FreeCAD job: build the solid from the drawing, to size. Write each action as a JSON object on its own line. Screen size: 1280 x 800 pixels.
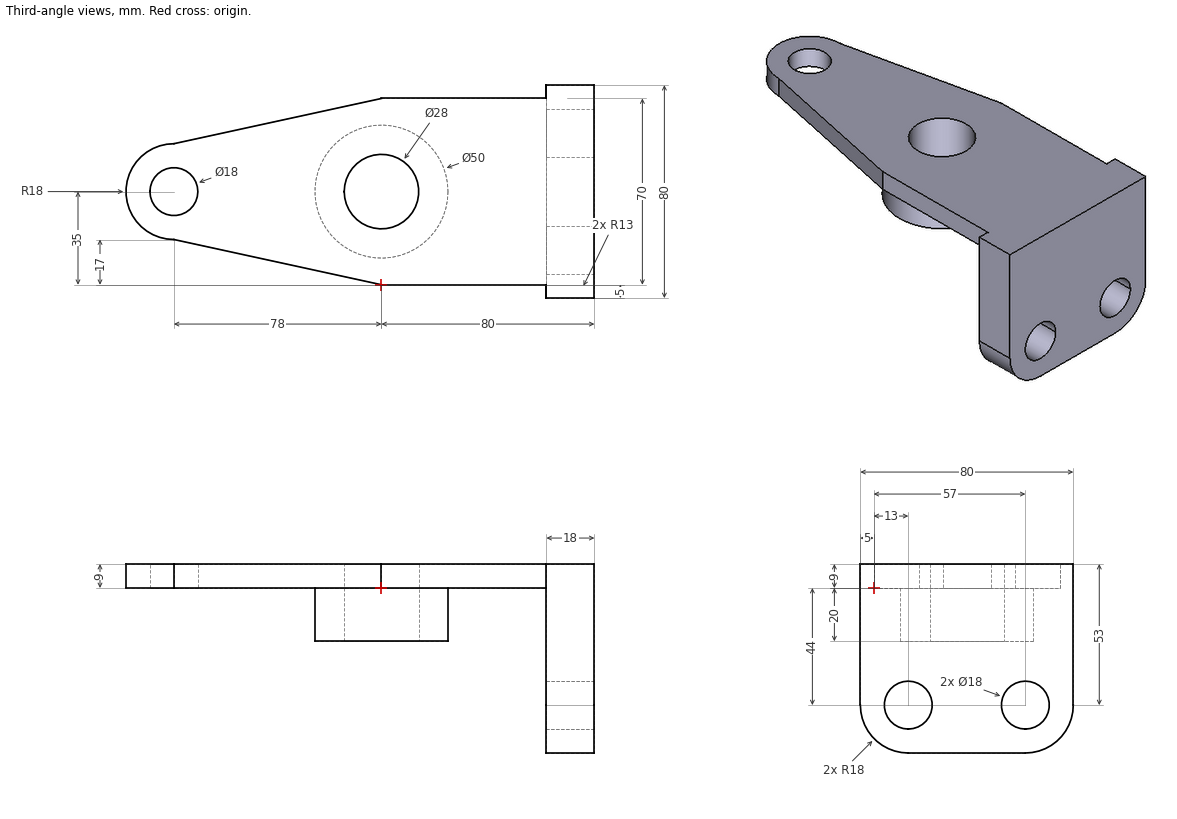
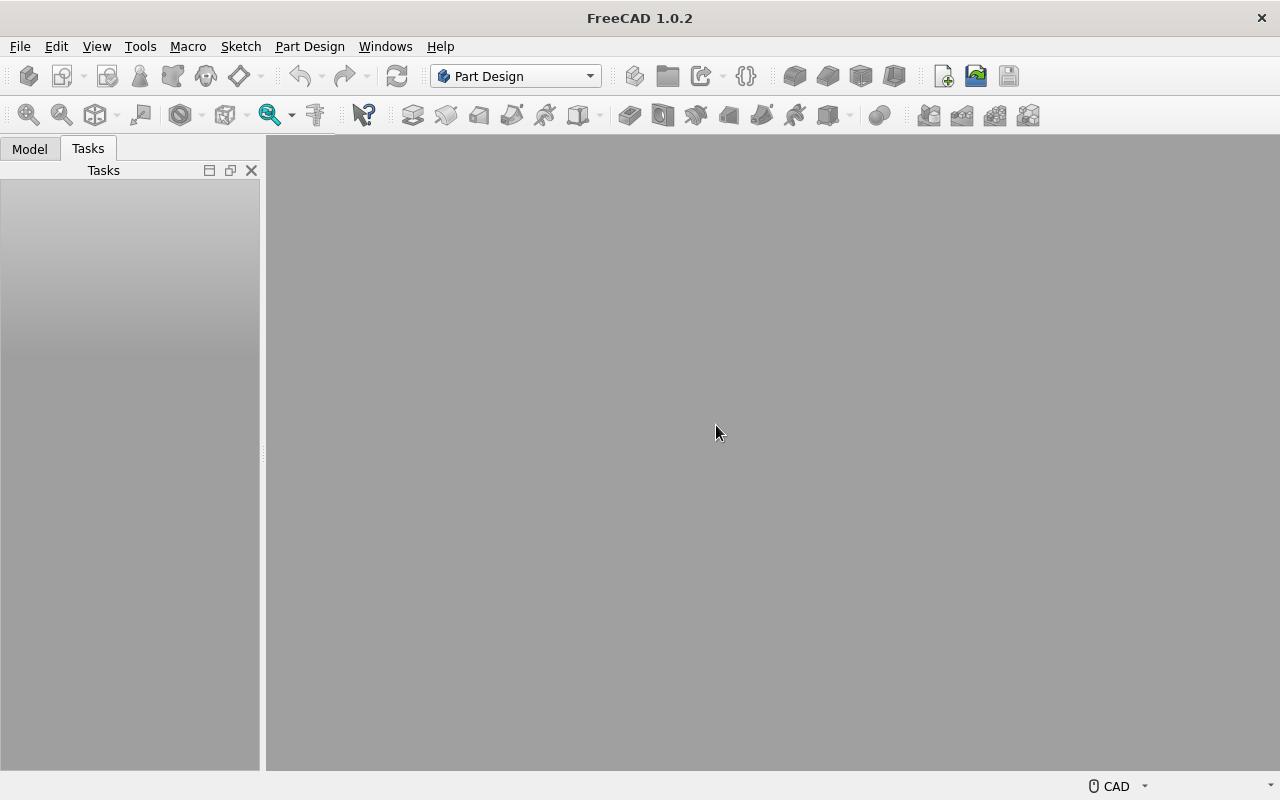
{"action": "left_click", "coordinate": [943, 76]}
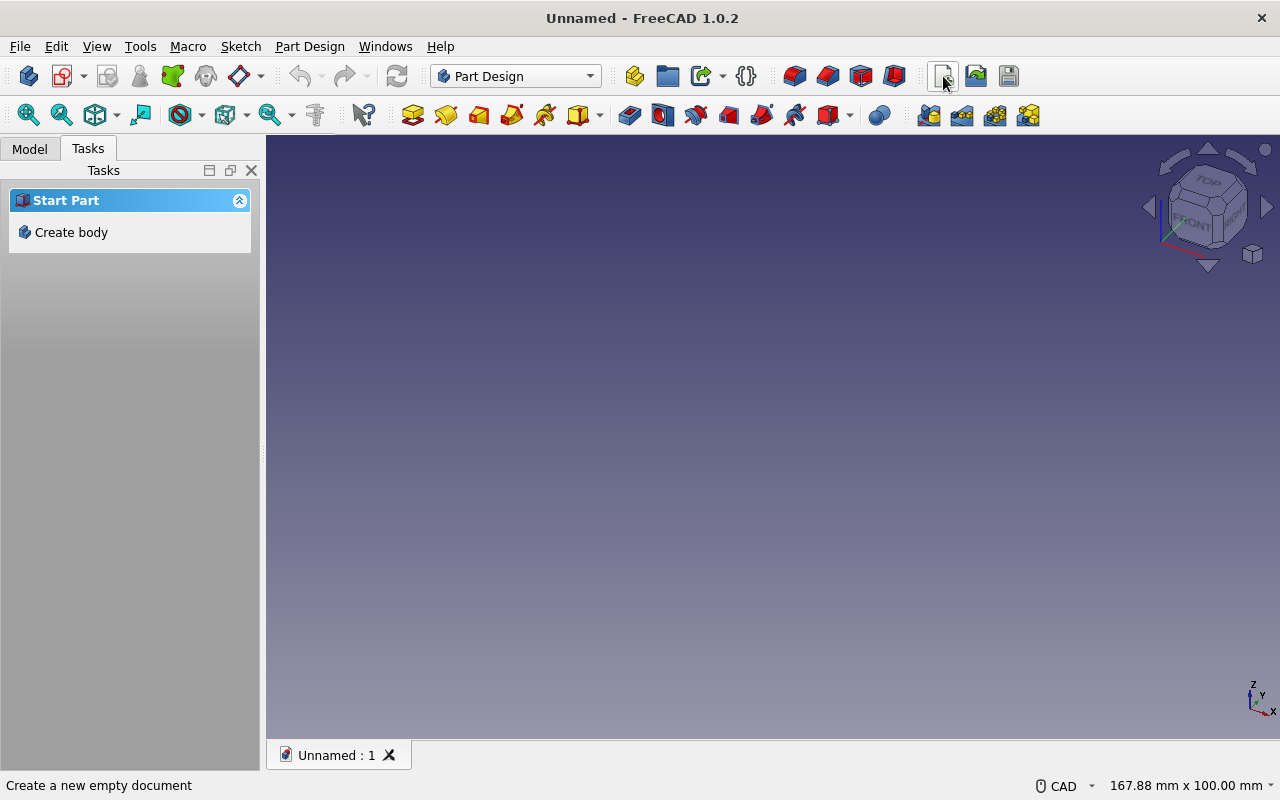
{"action": "left_click", "coordinate": [62, 76]}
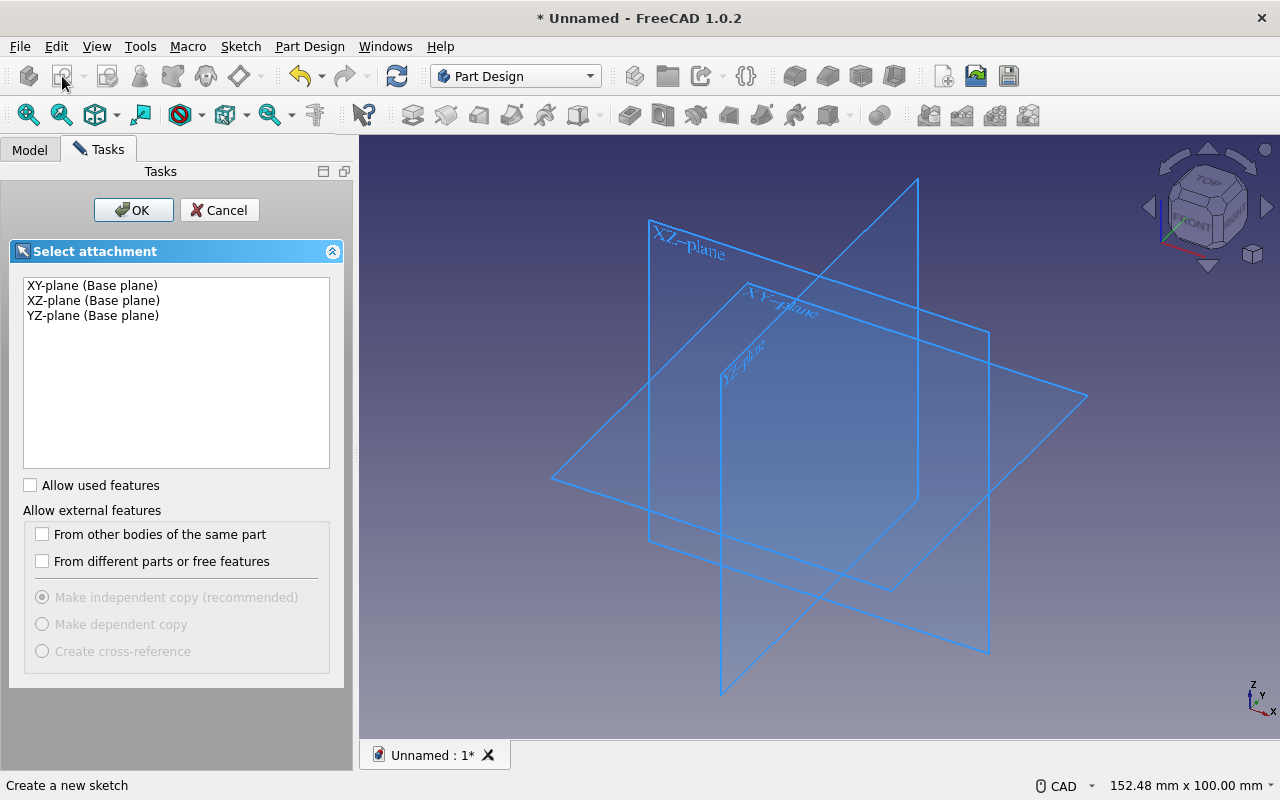
{"action": "left_click", "coordinate": [84, 286]}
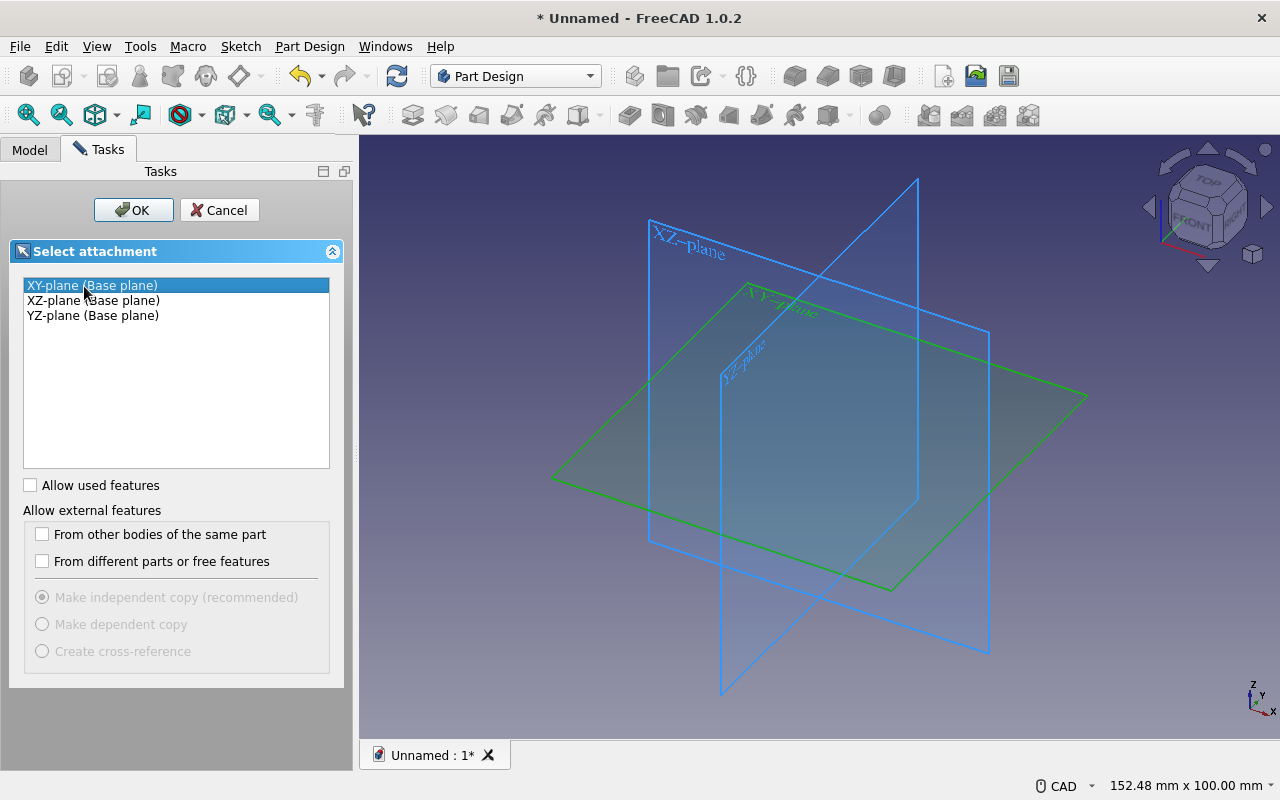
{"action": "left_click", "coordinate": [134, 210]}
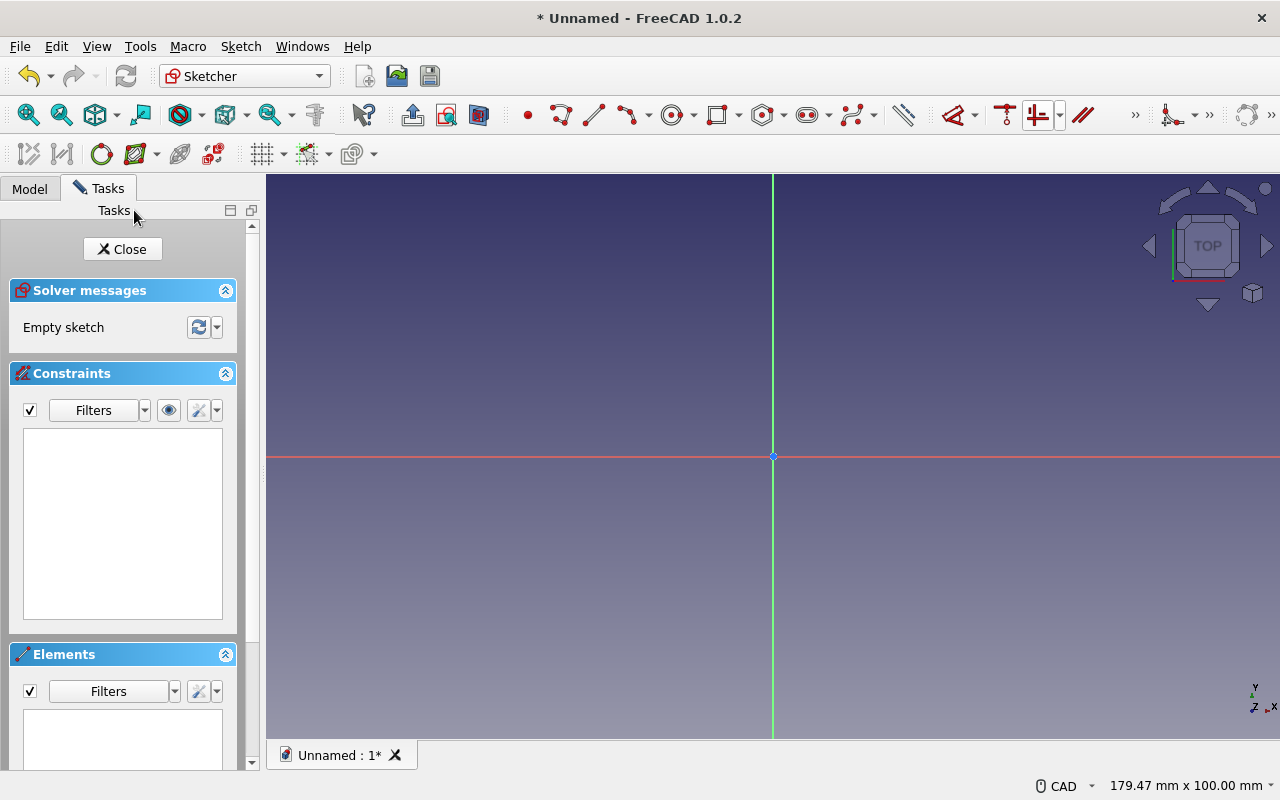
{"action": "scroll", "coordinate": [676, 697], "scroll_direction": "down", "scroll_amount": 3}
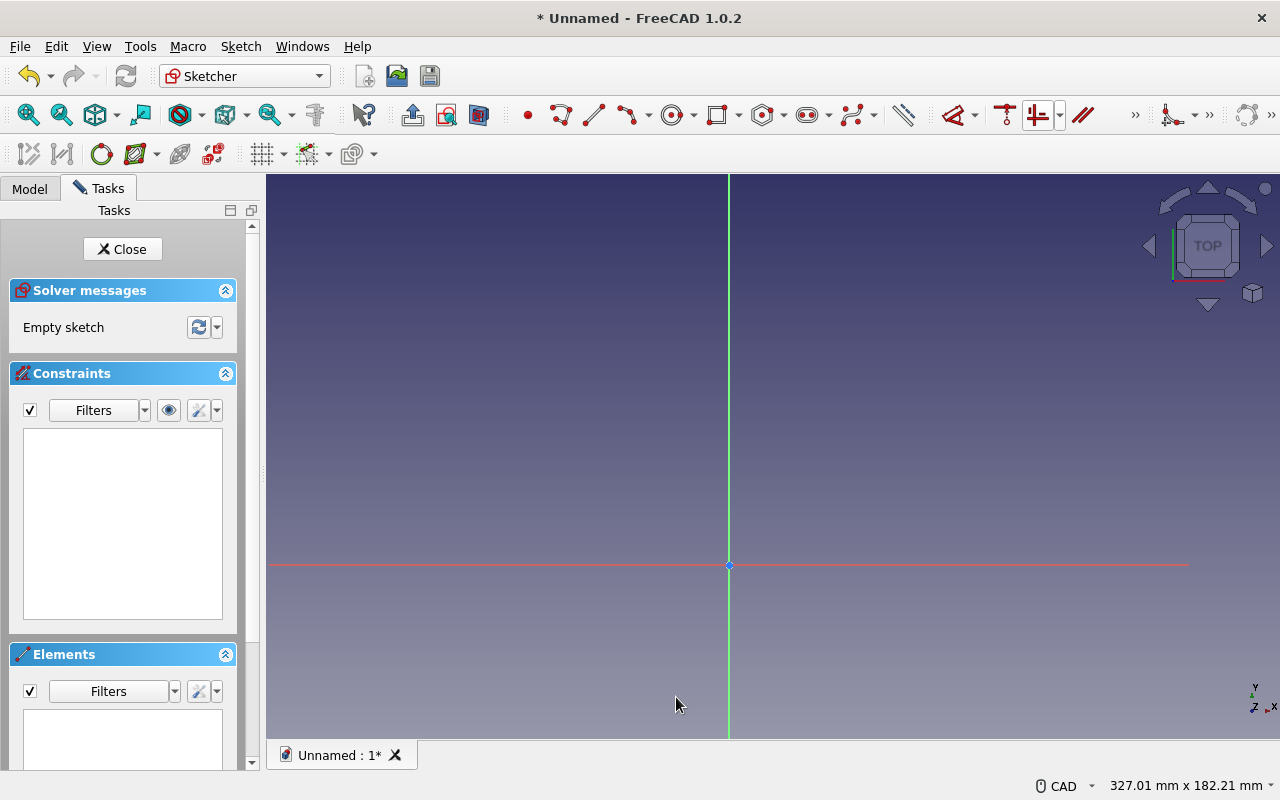
{"action": "left_click", "coordinate": [561, 116]}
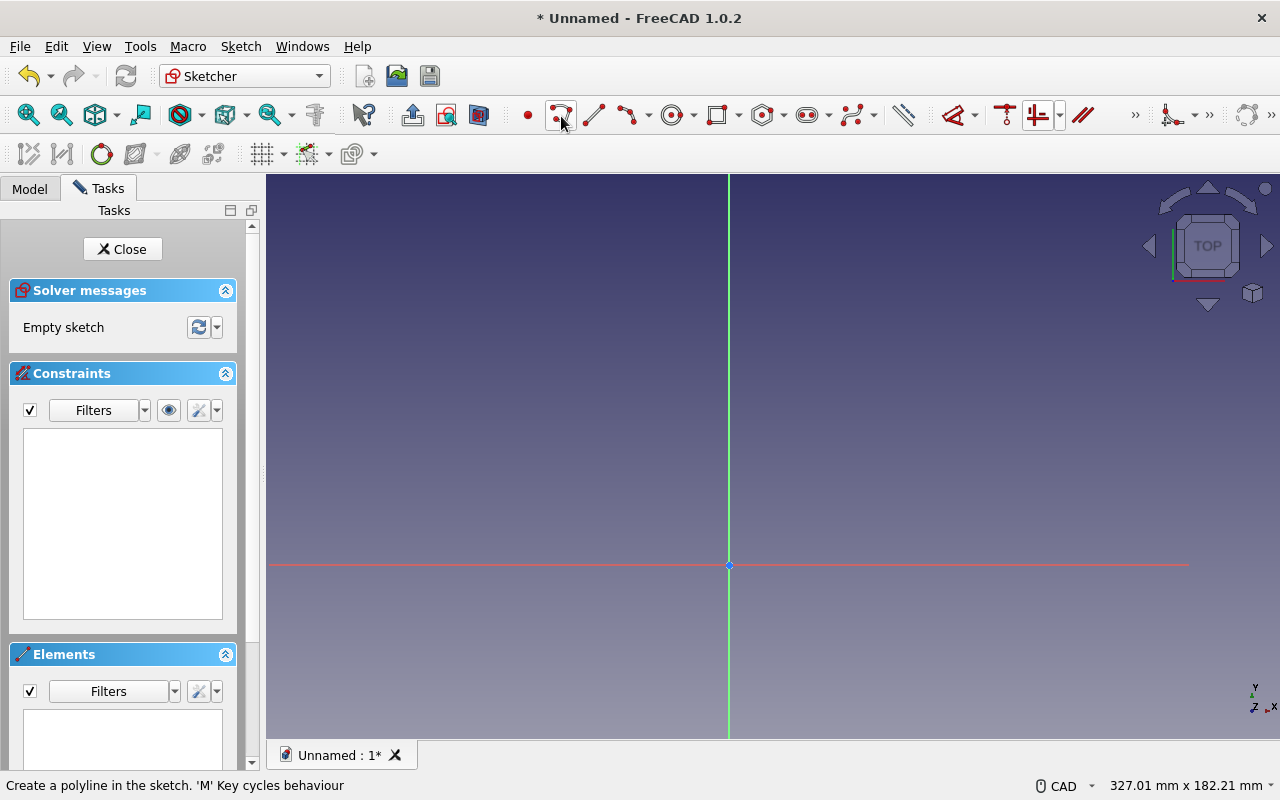
{"action": "left_click", "coordinate": [488, 513]}
{"action": "left_click", "coordinate": [729, 565]}
{"action": "left_click", "coordinate": [946, 556]}
{"action": "right_click", "coordinate": [946, 556]}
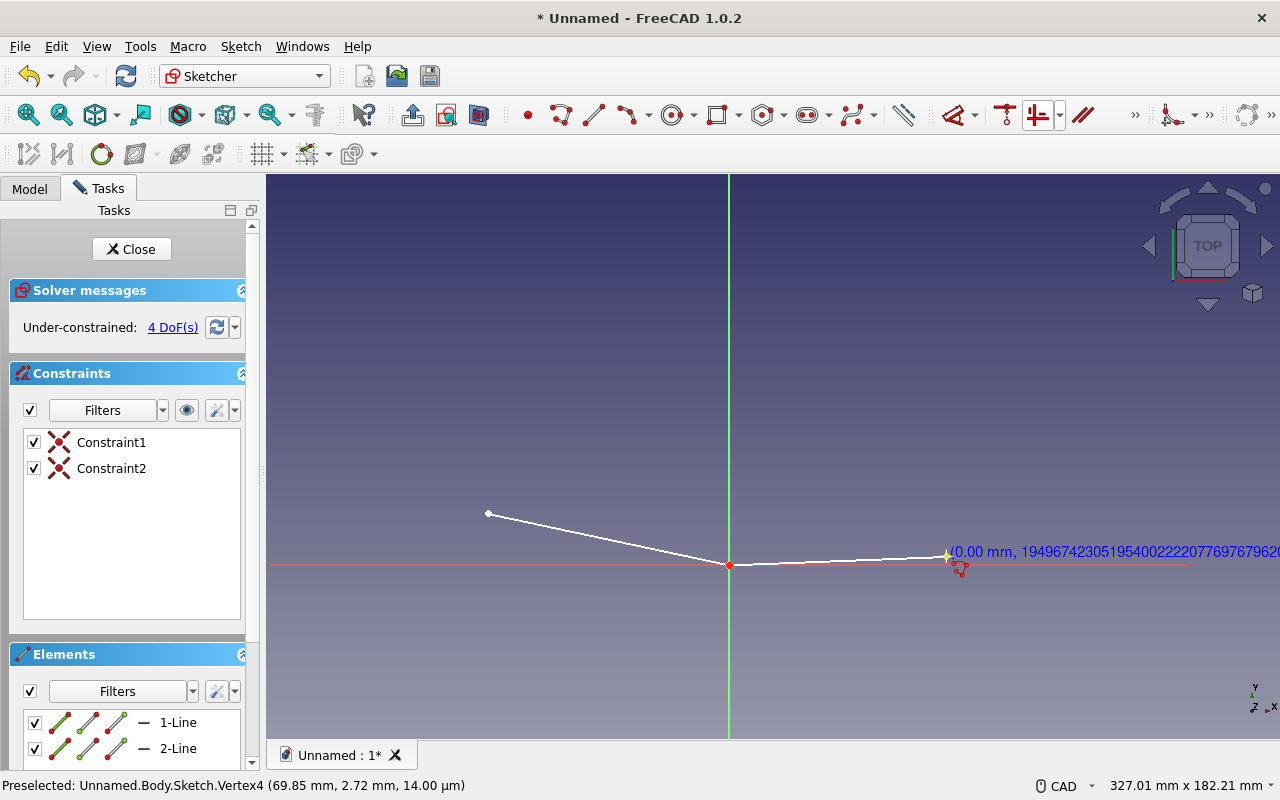
{"action": "left_click", "coordinate": [594, 116]}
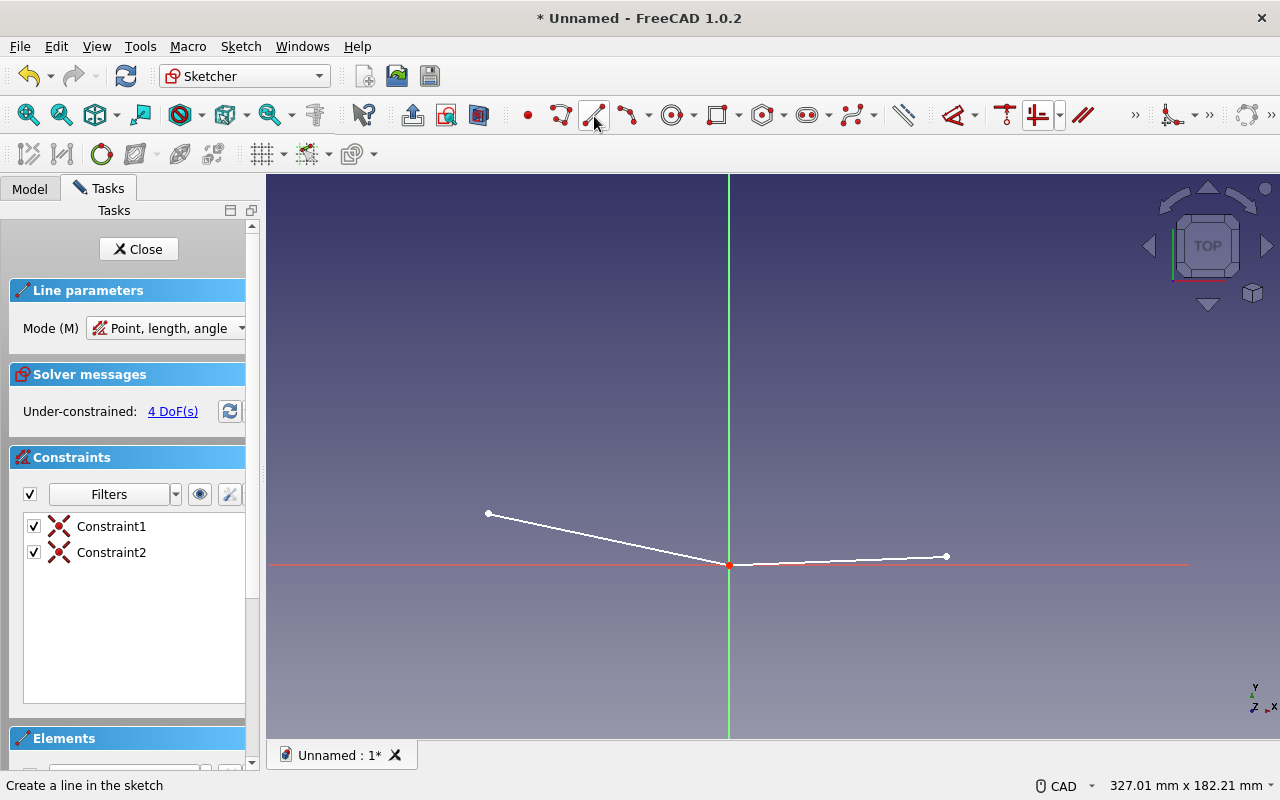
{"action": "left_click", "coordinate": [977, 581]}
{"action": "left_click", "coordinate": [977, 333]}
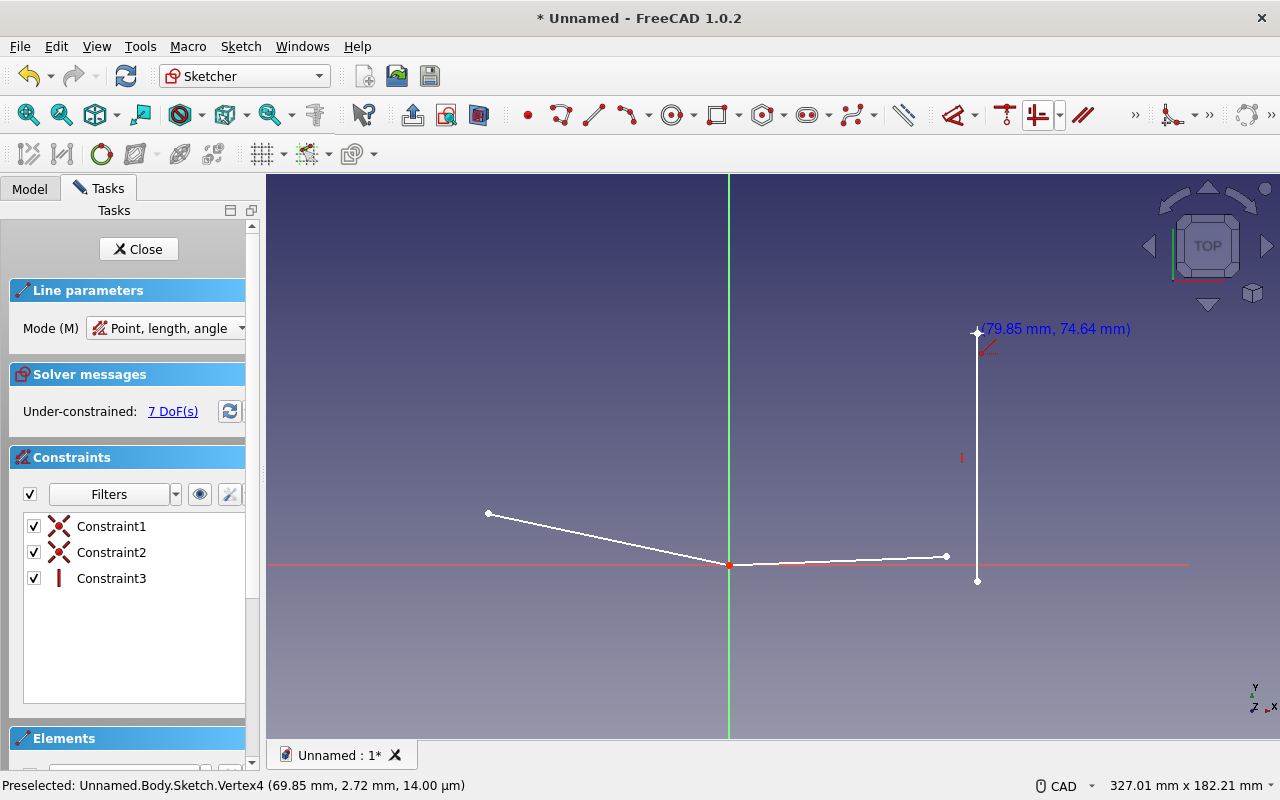
{"action": "left_click", "coordinate": [561, 116]}